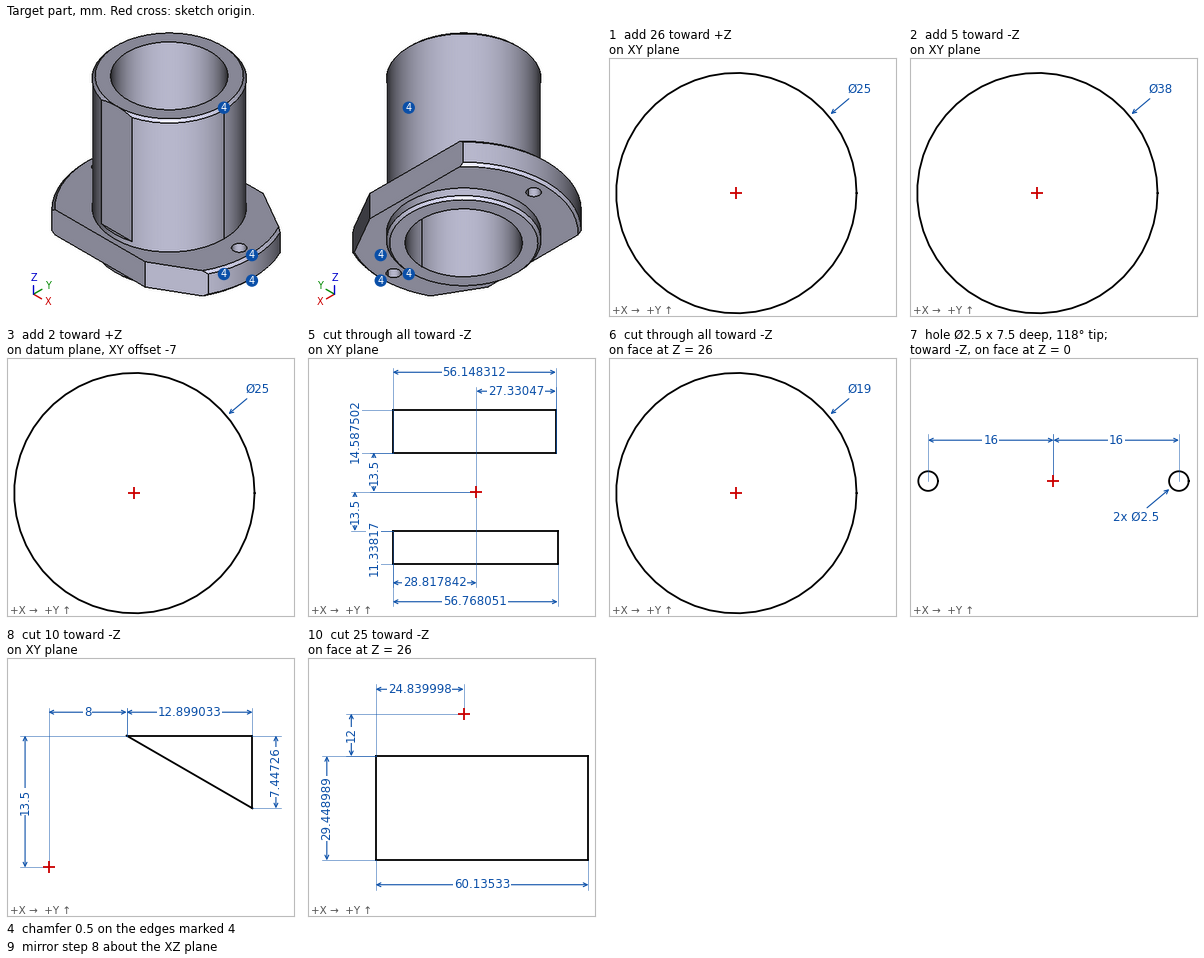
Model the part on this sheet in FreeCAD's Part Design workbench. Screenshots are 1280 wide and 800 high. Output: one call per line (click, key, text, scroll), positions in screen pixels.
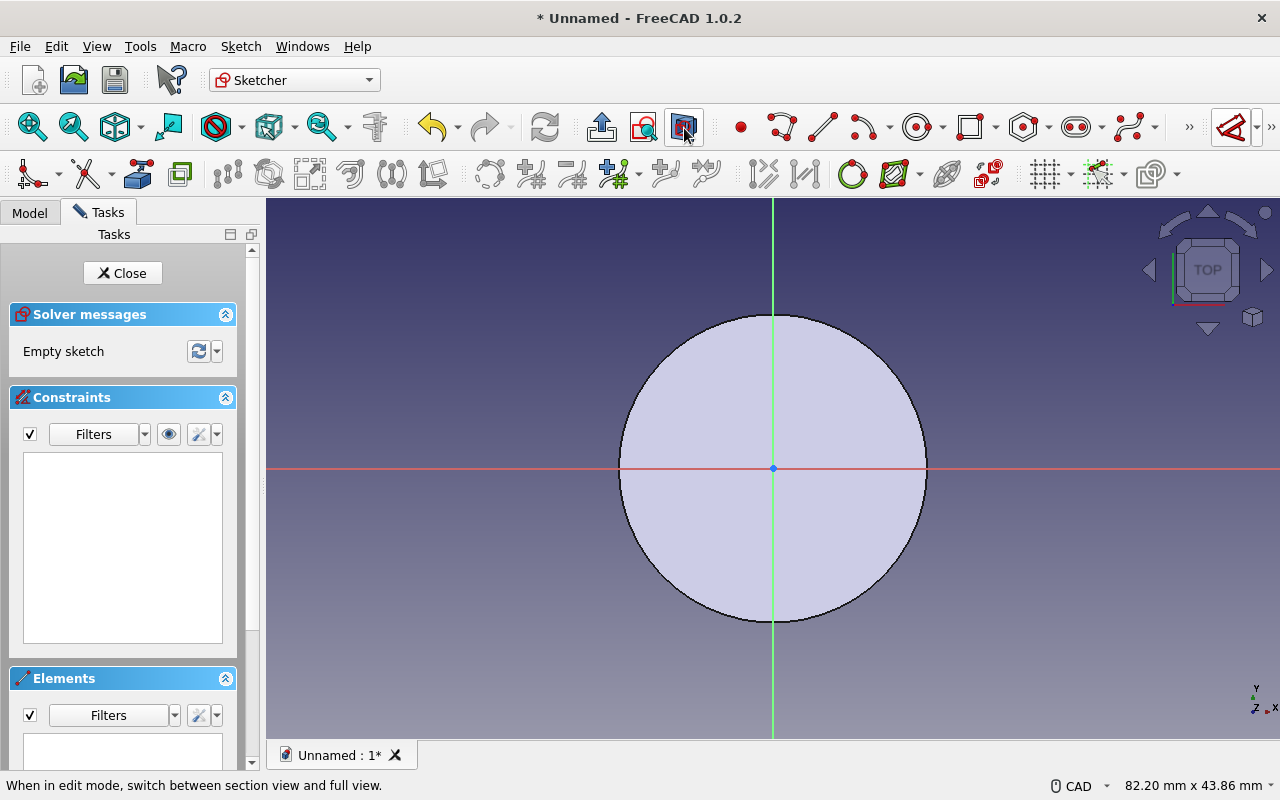
scroll(565, 468, down, 2)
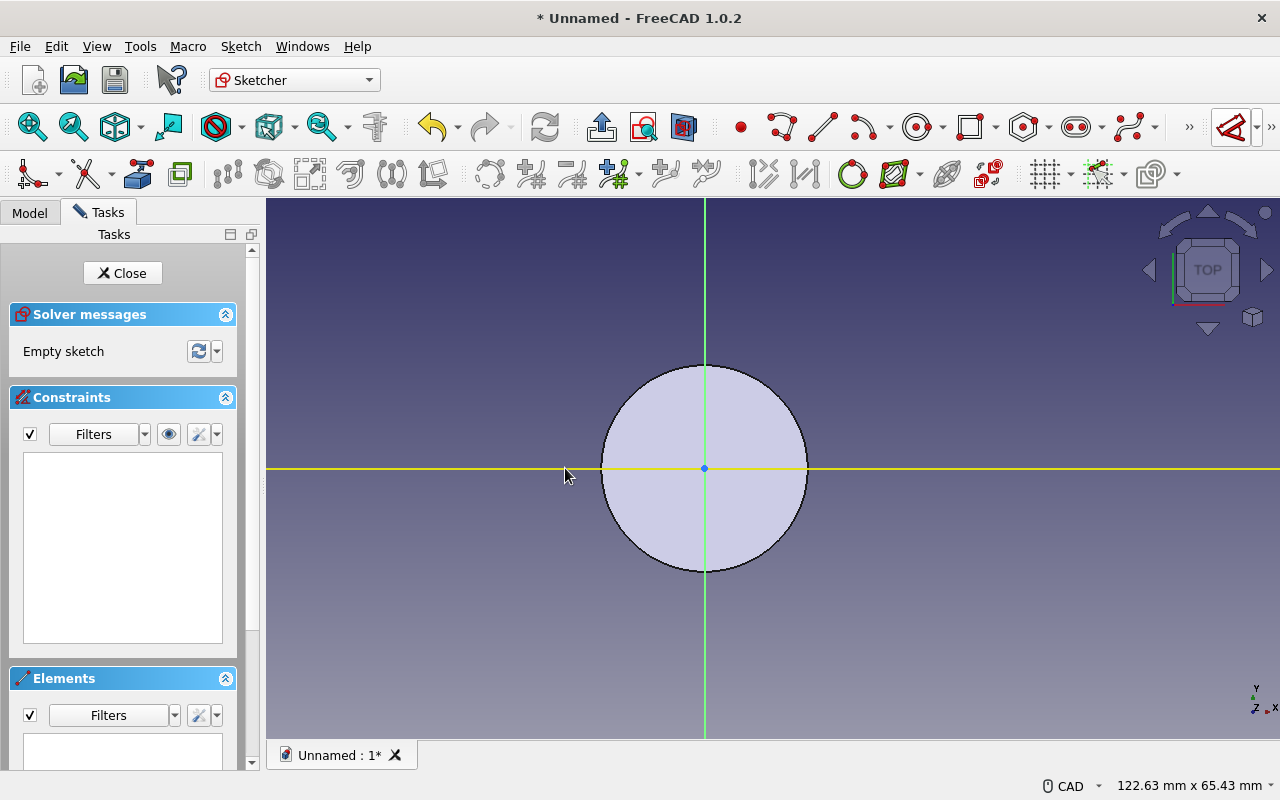
click(916, 128)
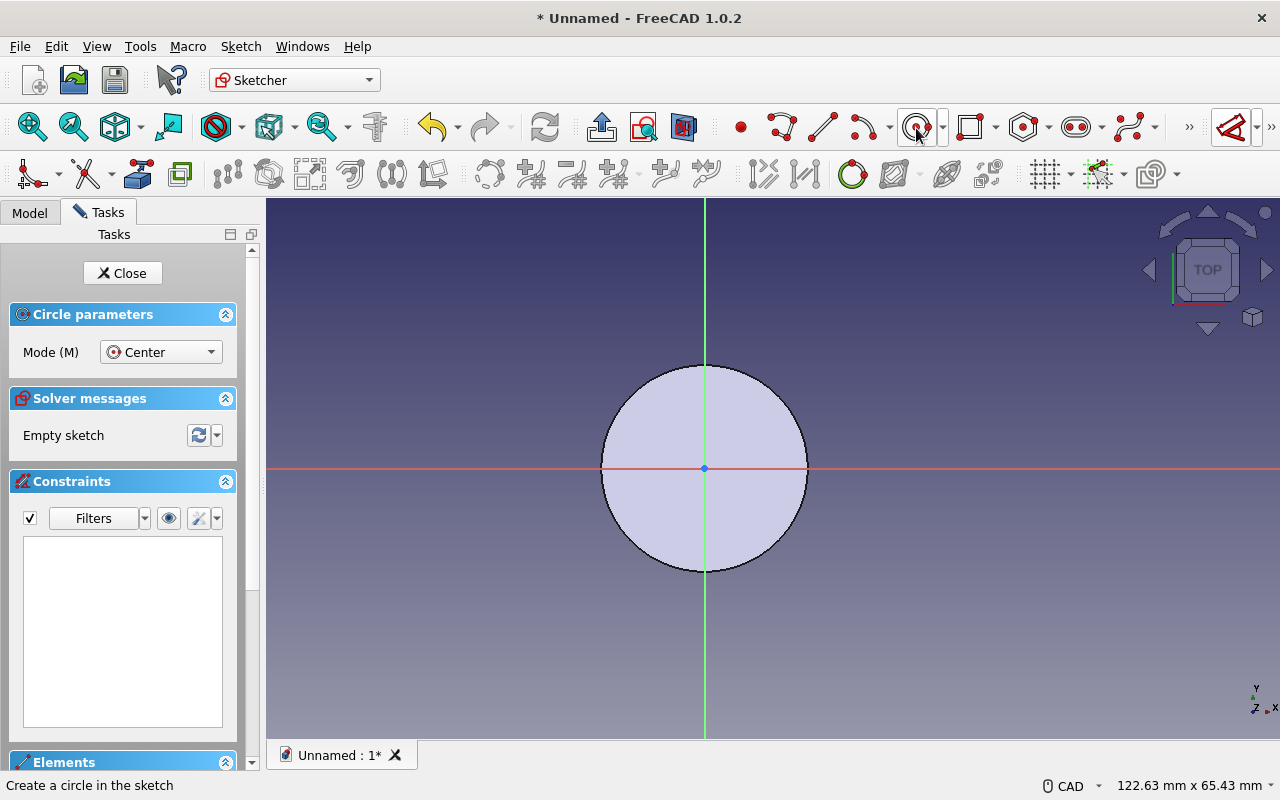
click(705, 468)
click(816, 357)
key(Escape)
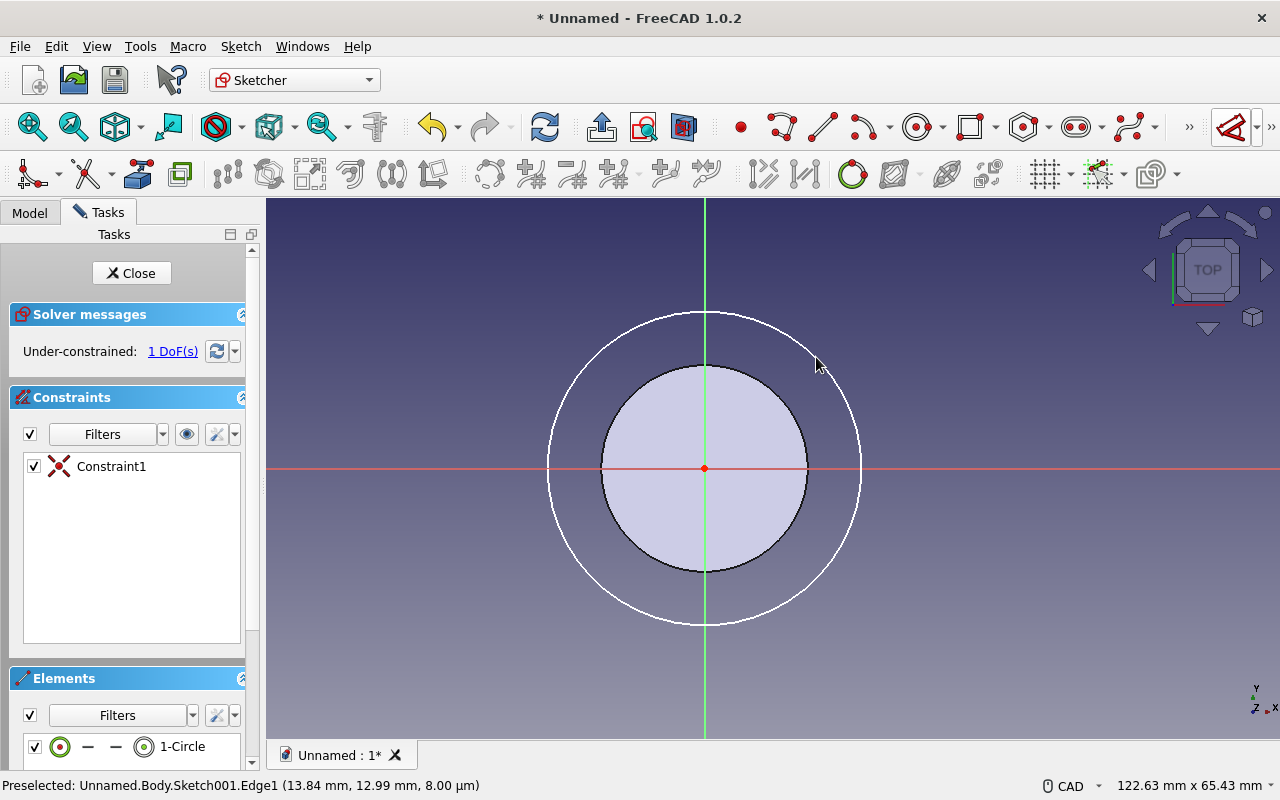
click(815, 357)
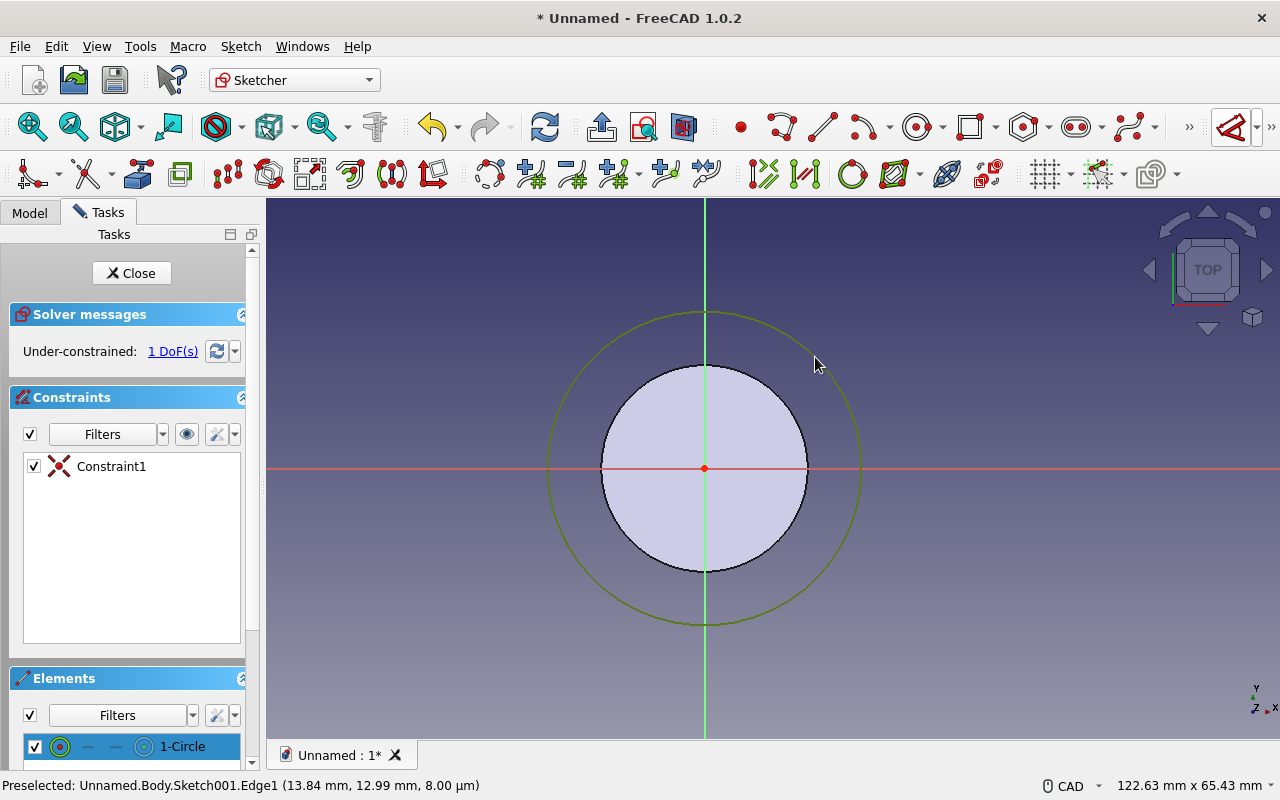
key(k)
key(o)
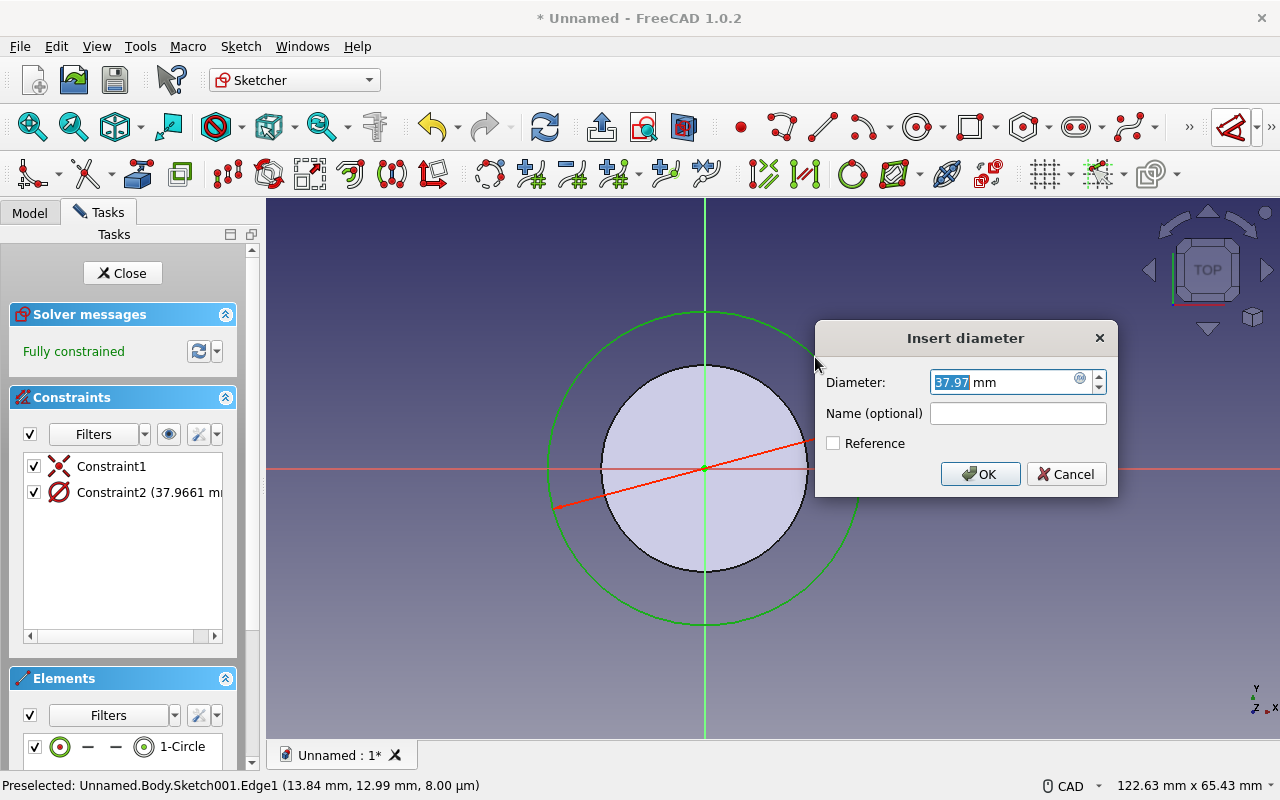
text(38)
key(Return)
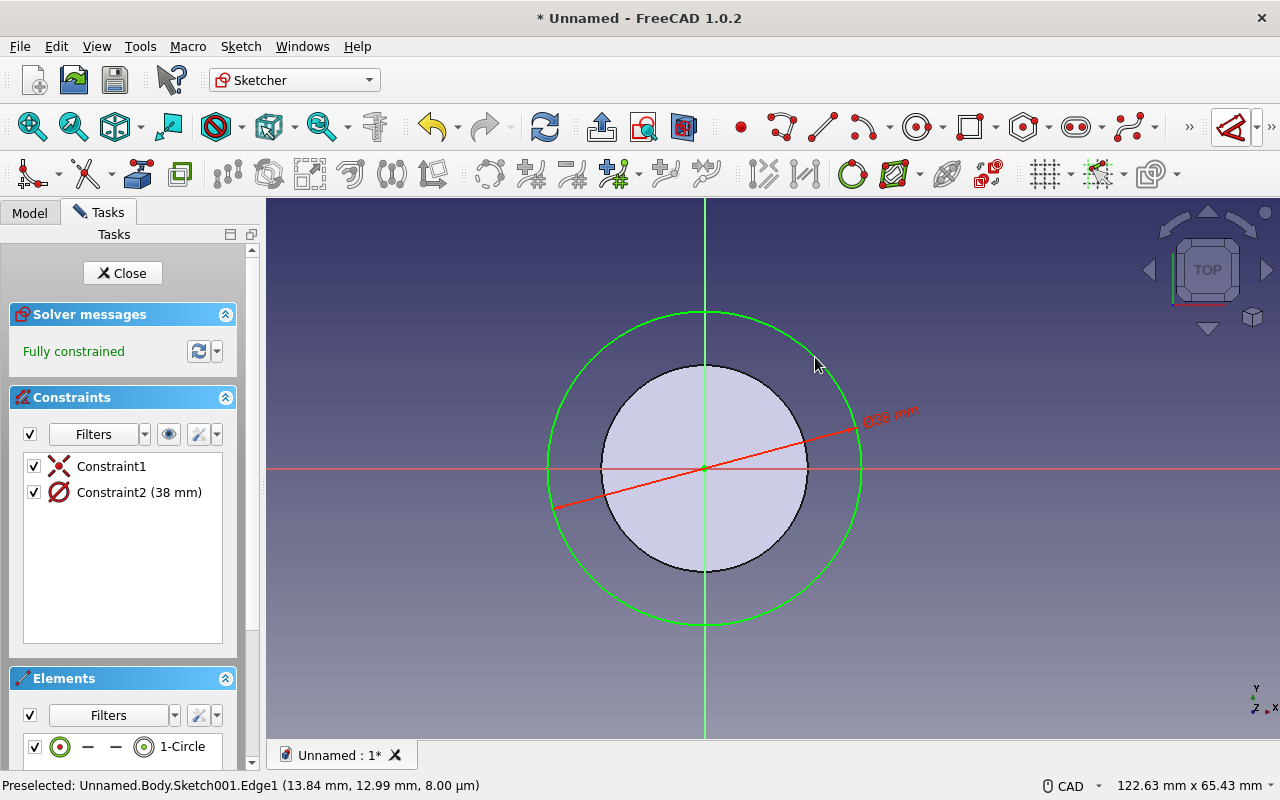
click(123, 273)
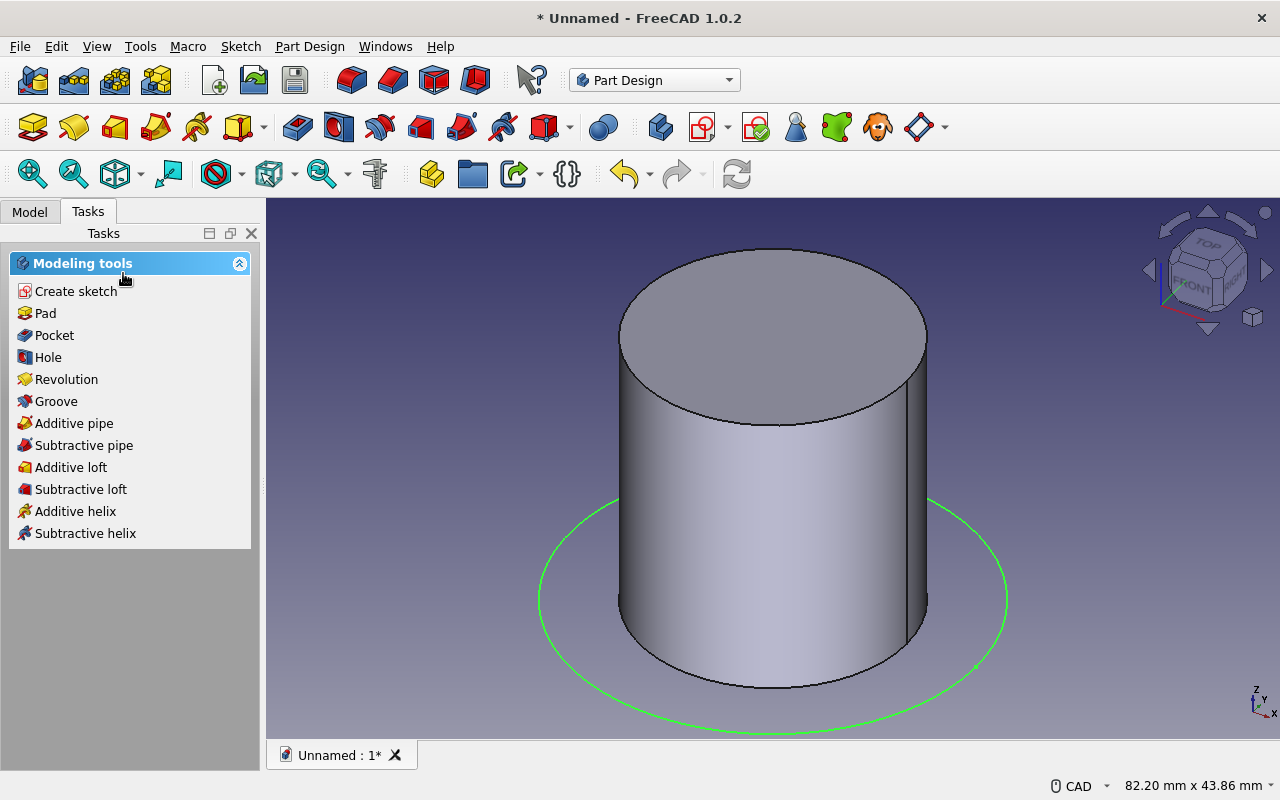
click(33, 128)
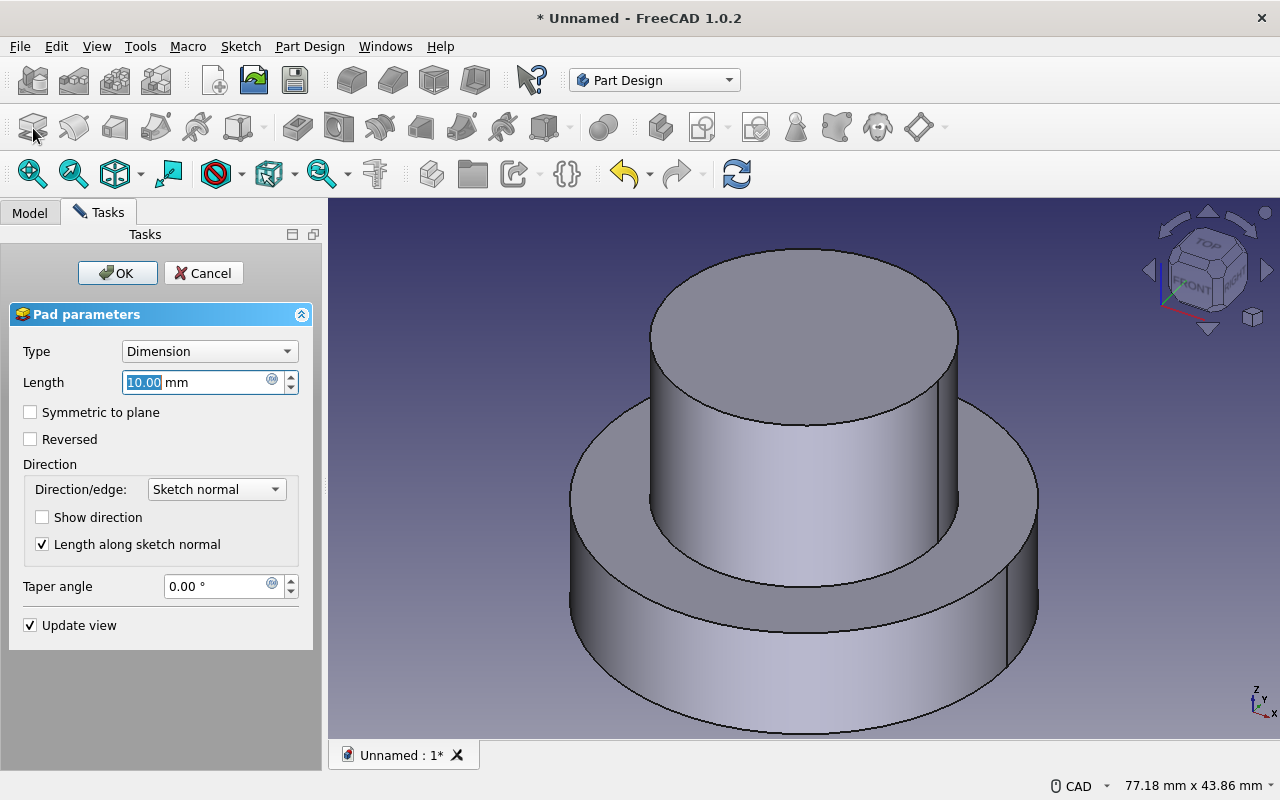
text(5)
key(Tab)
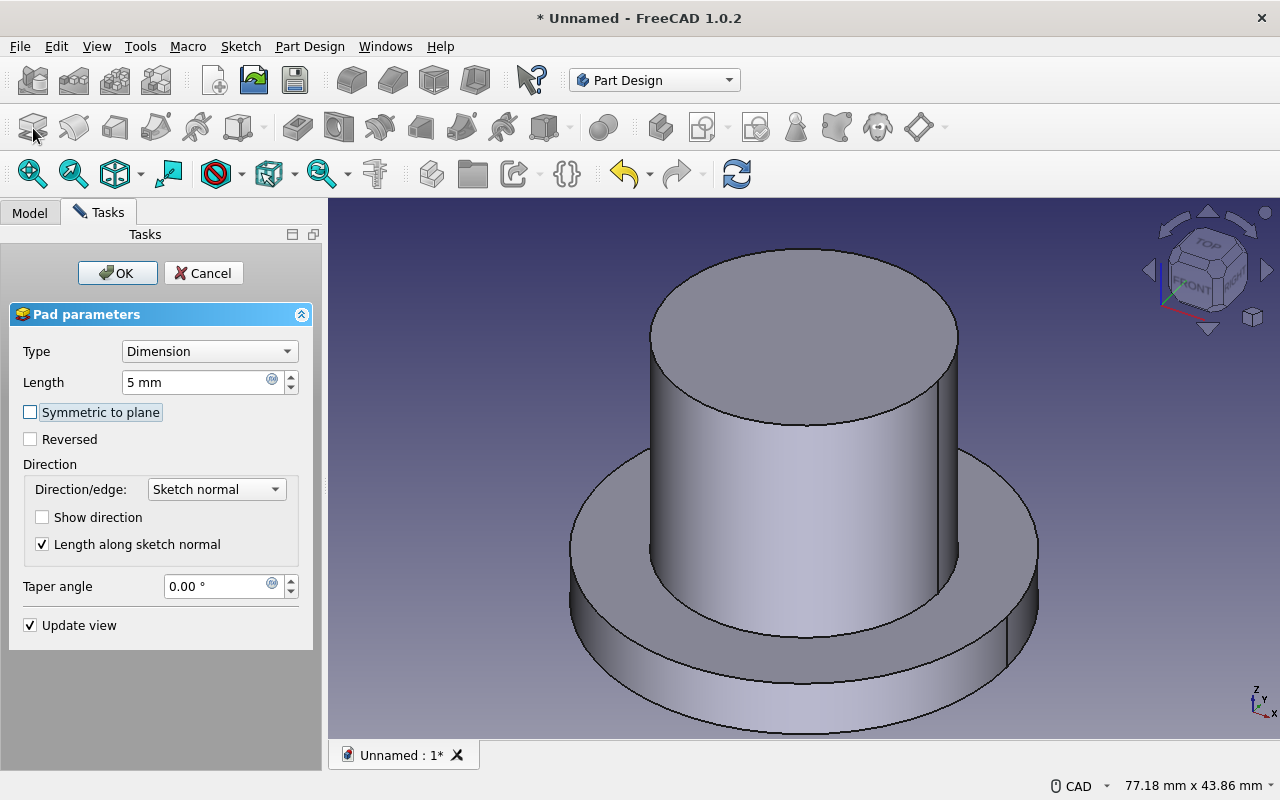
click(31, 439)